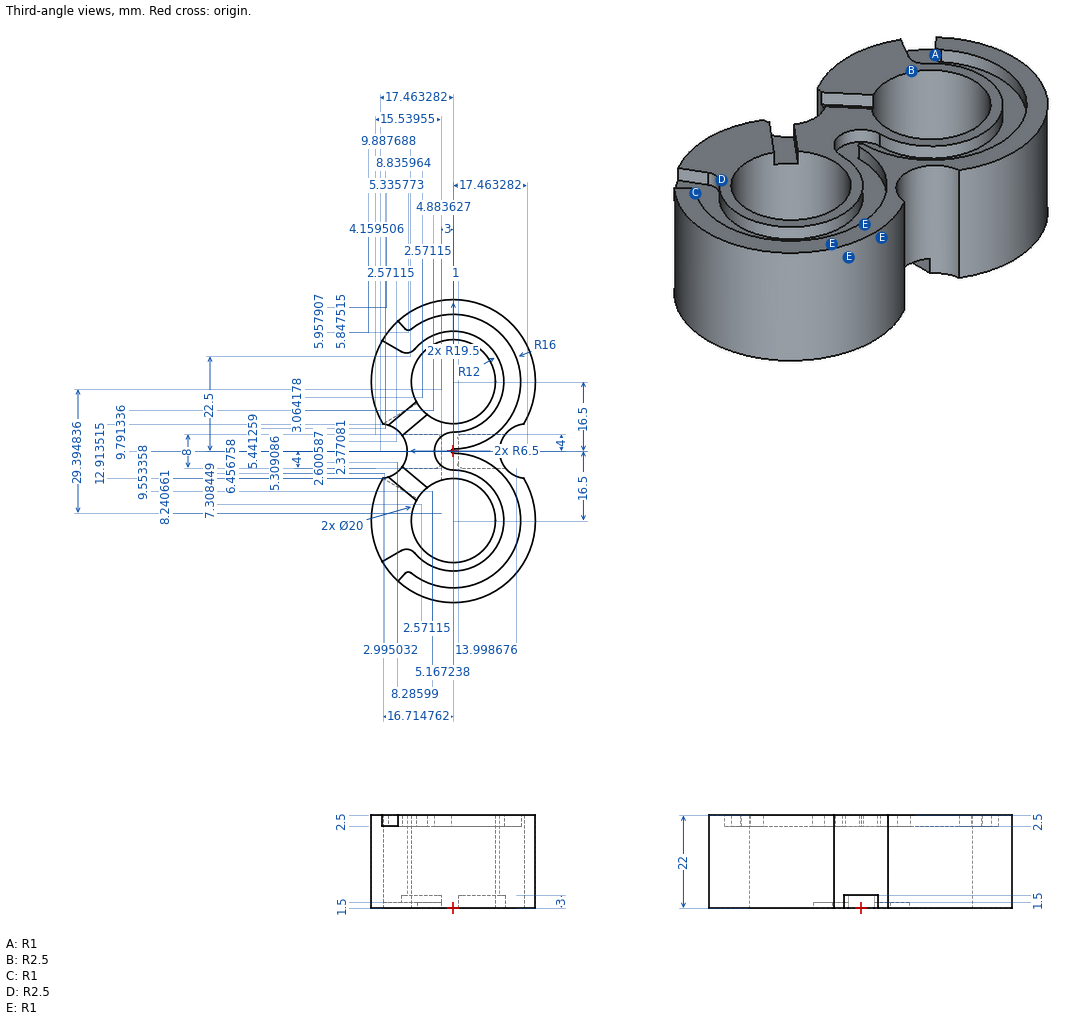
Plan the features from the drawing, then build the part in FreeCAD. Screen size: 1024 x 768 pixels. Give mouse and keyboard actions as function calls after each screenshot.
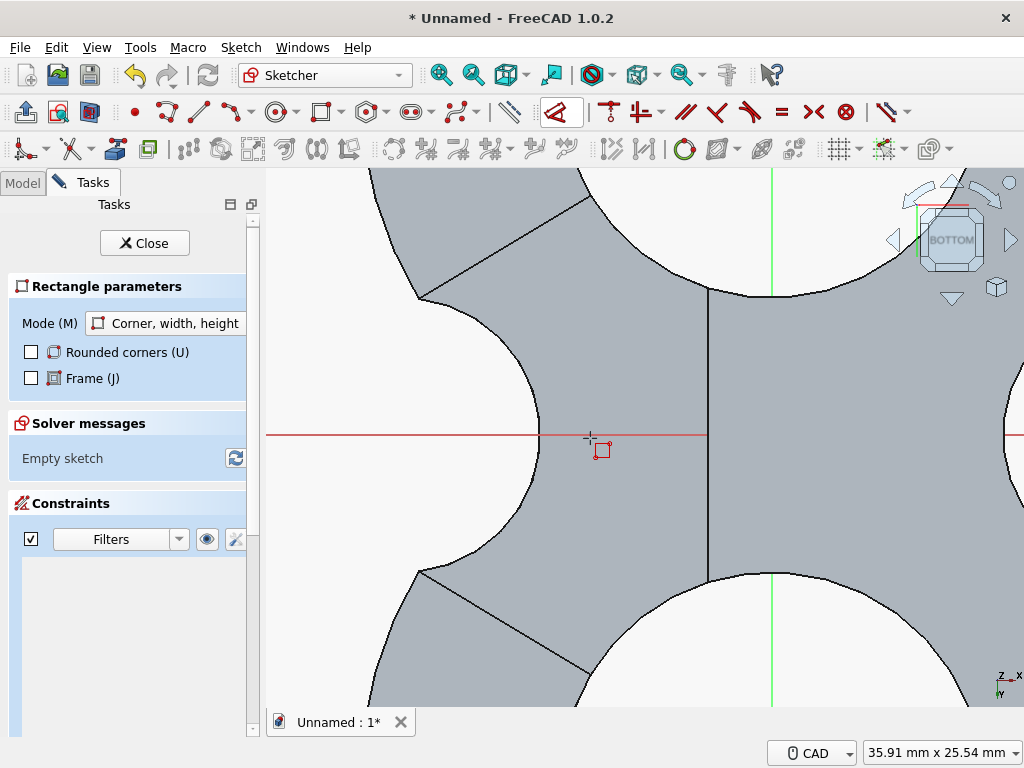
click(380, 351)
move(708, 520)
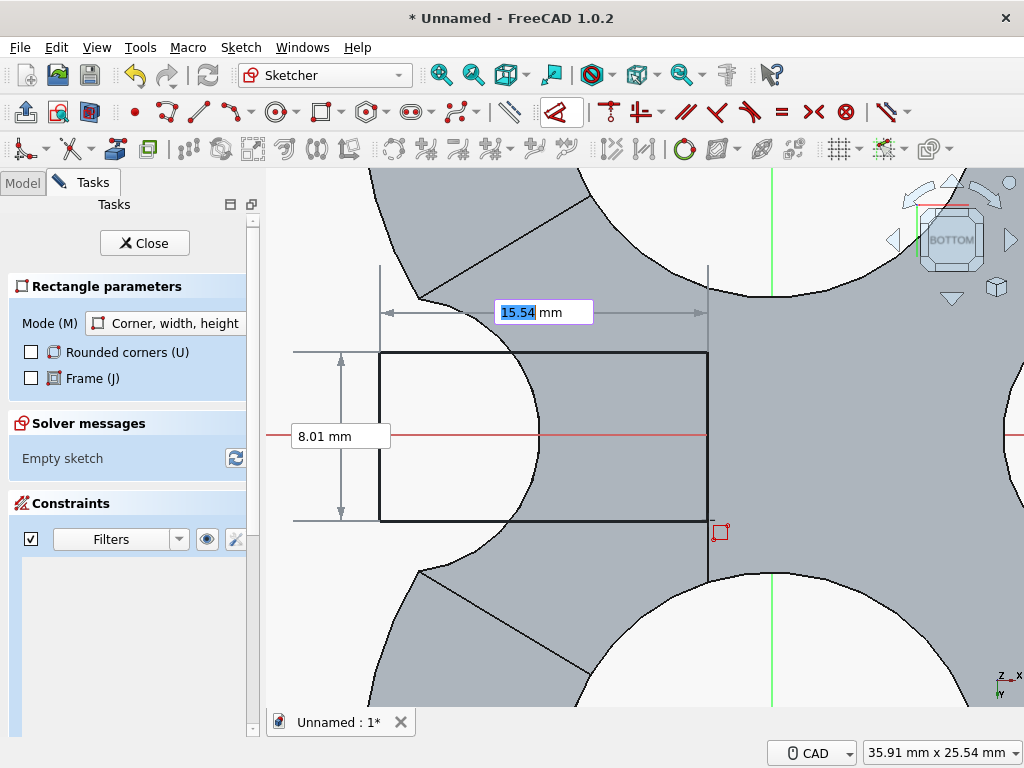
text(15.53955)
key(Tab)
text(8)
key(Return)
key(Escape)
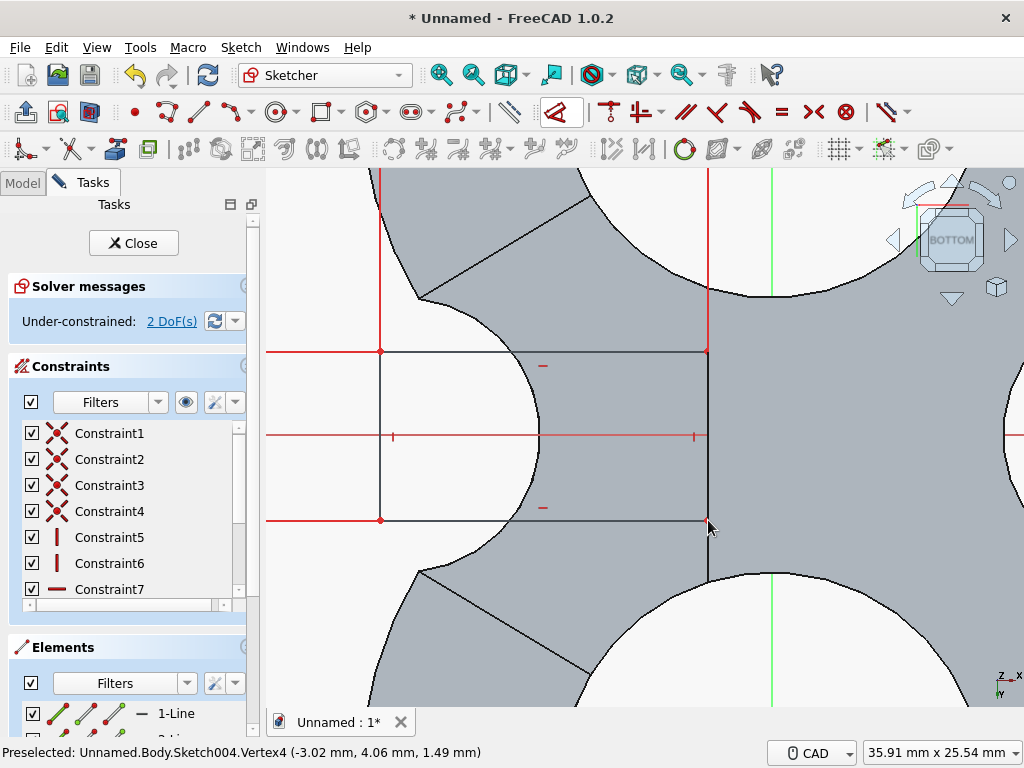
click(380, 352)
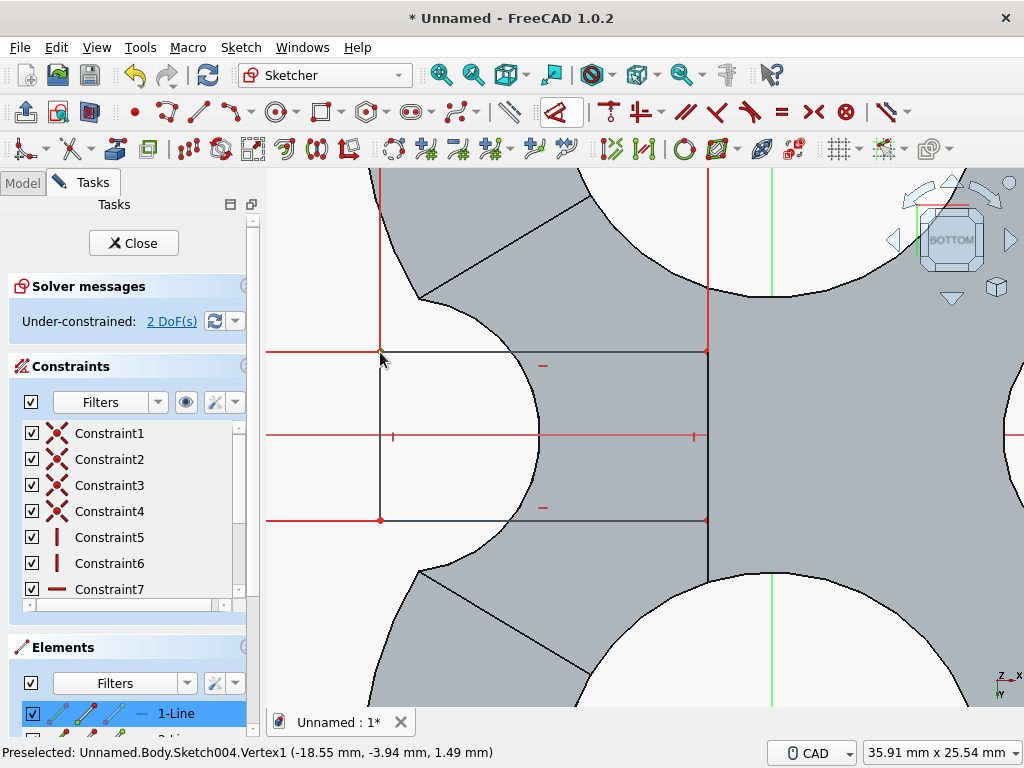
key(i)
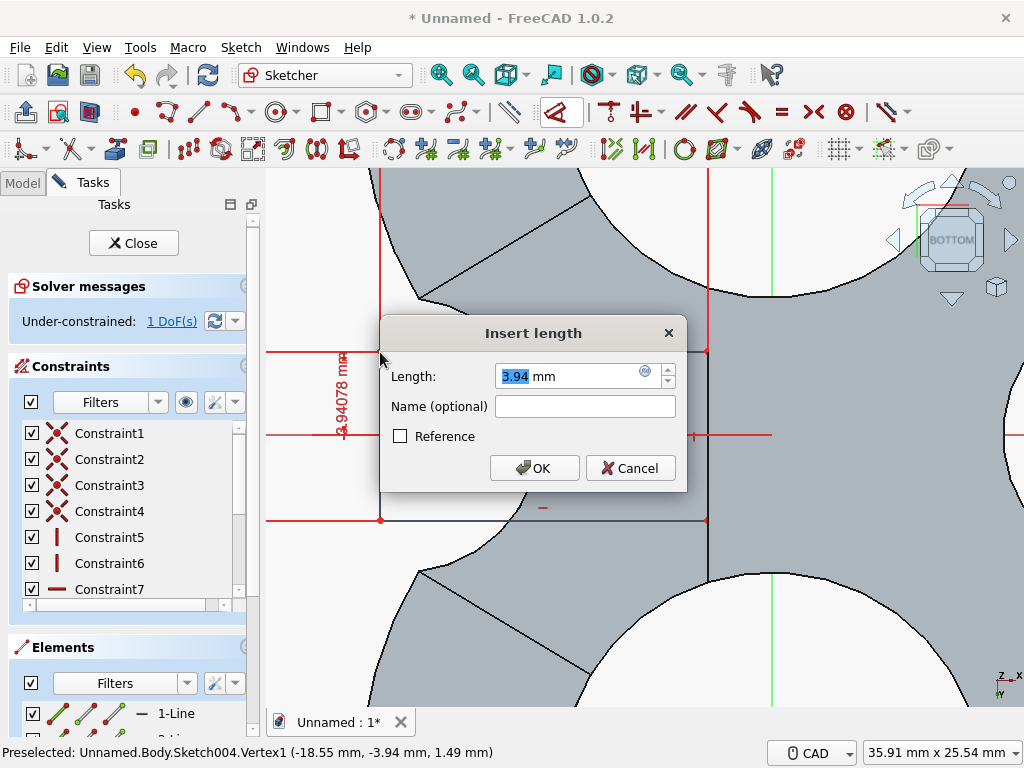
text(4)
key(Return)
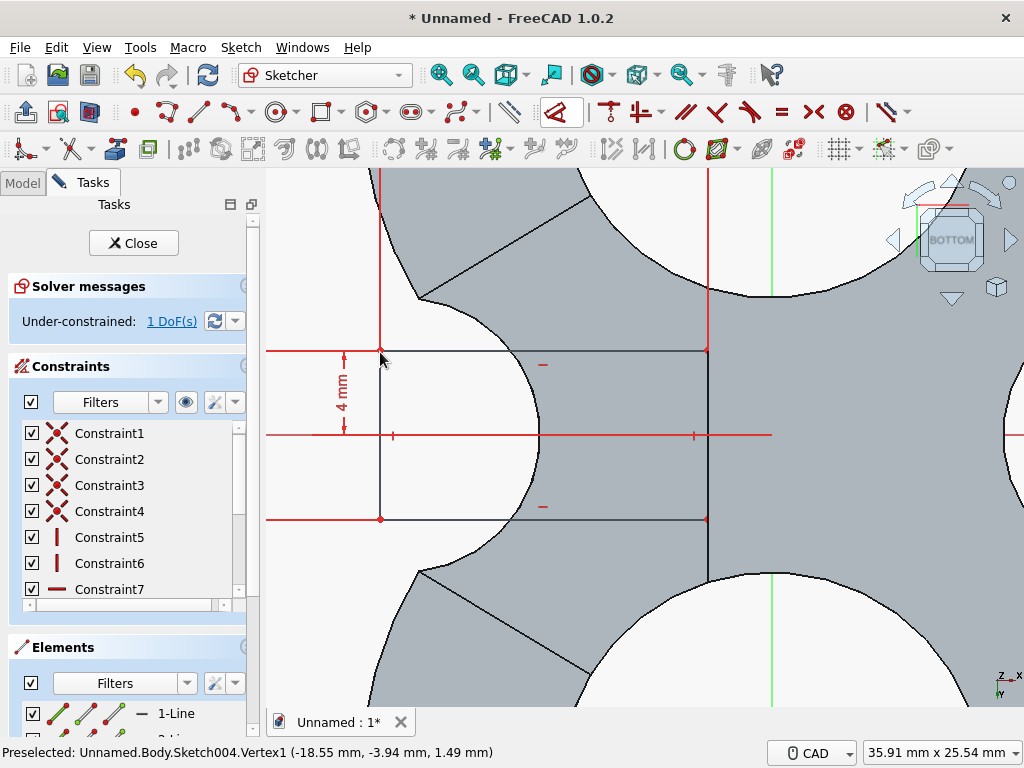
click(708, 520)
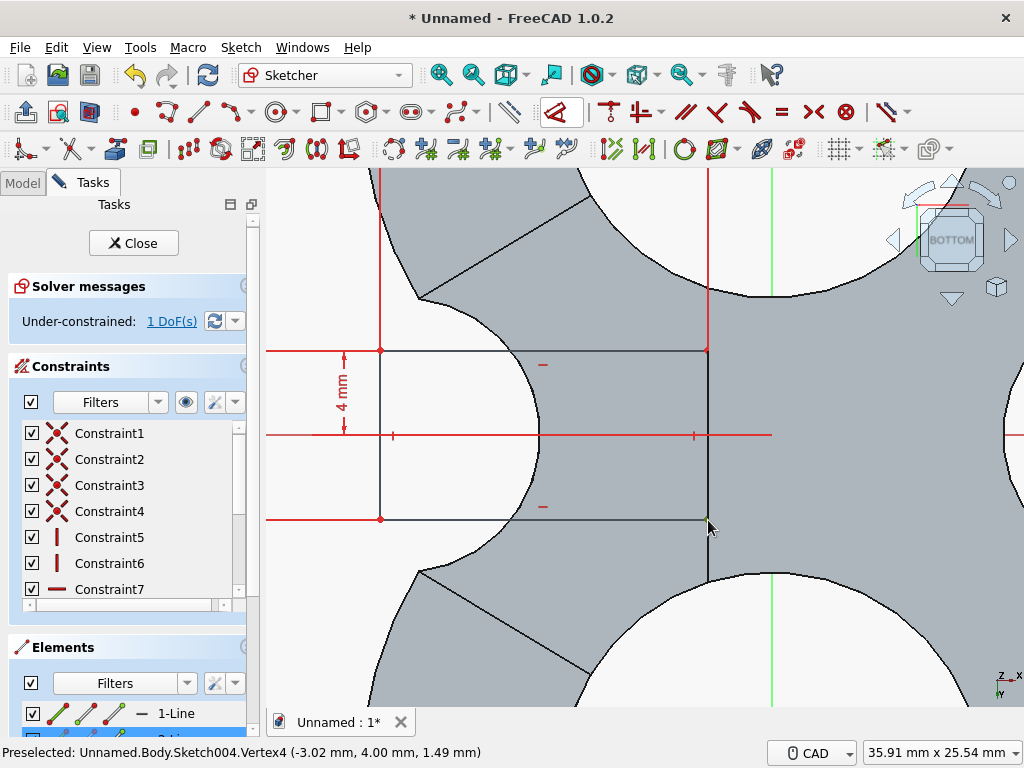
key(l)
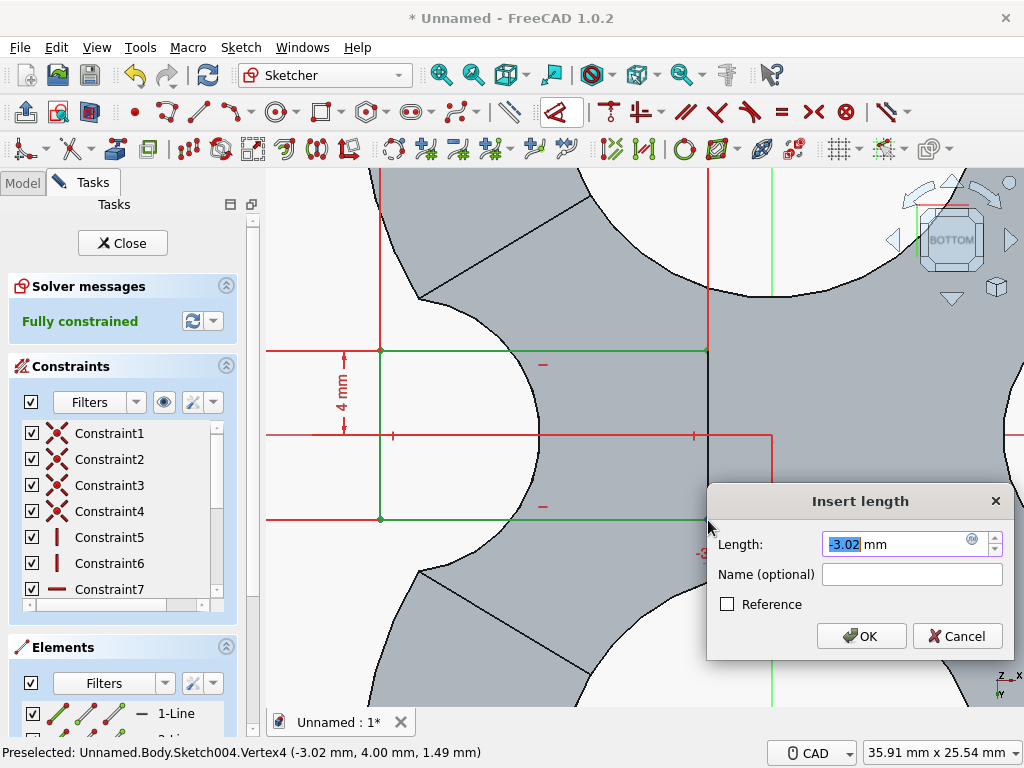
text(-3)
key(Return)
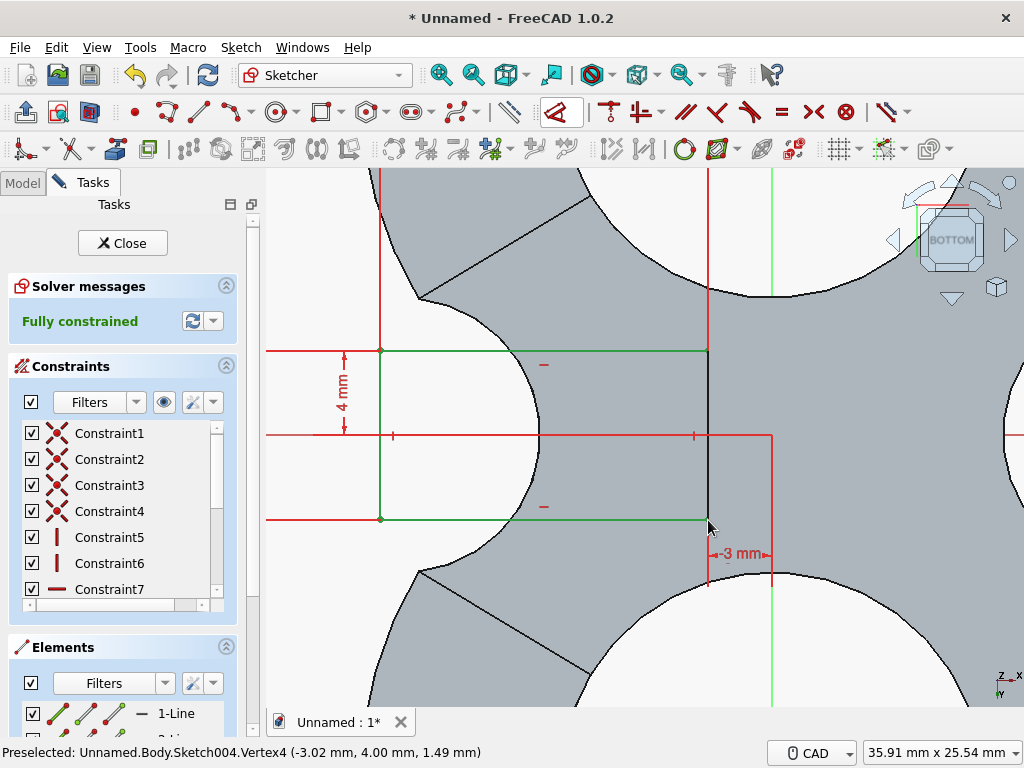
click(123, 243)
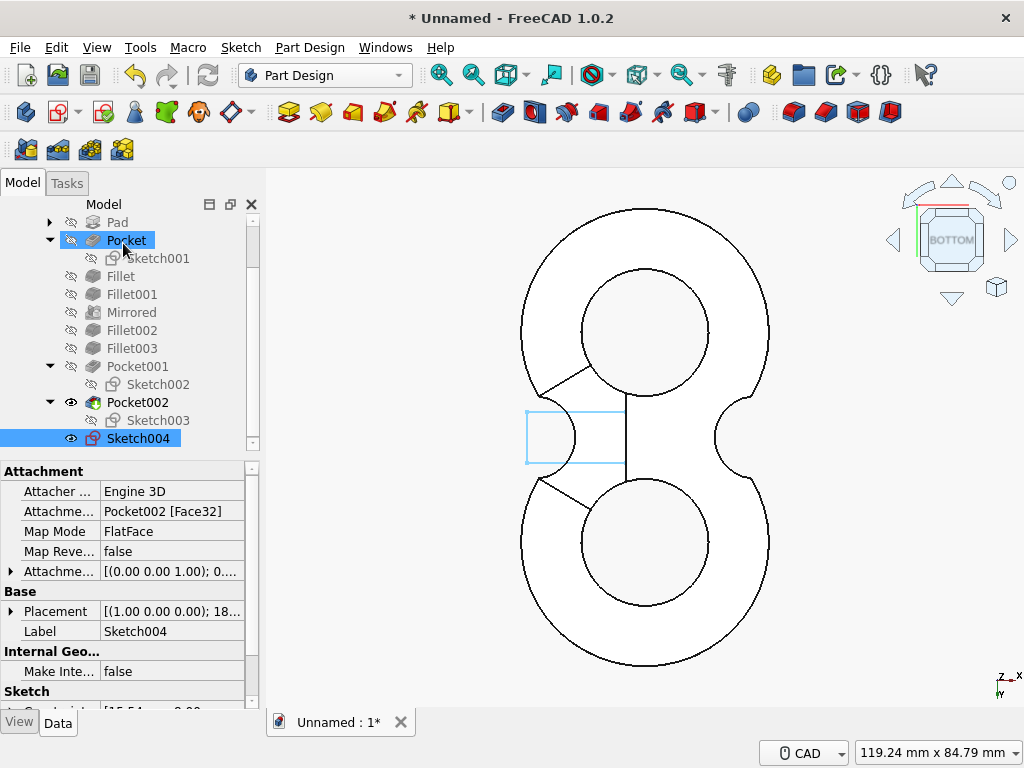
click(504, 112)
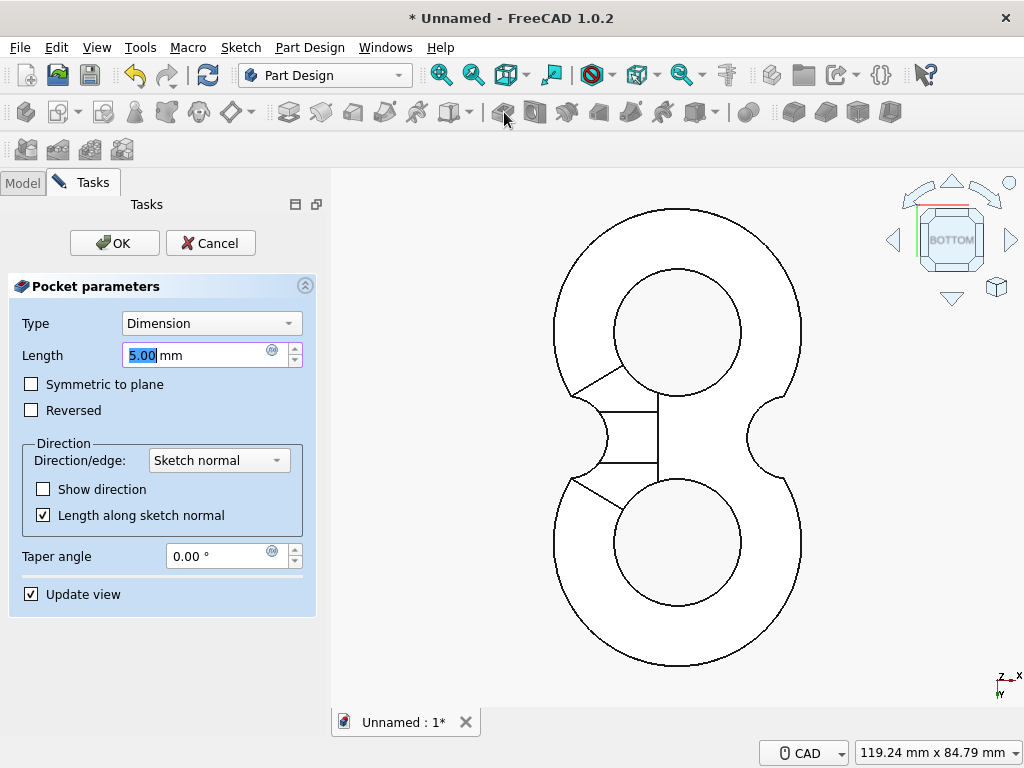
text(1.5)
key(Tab)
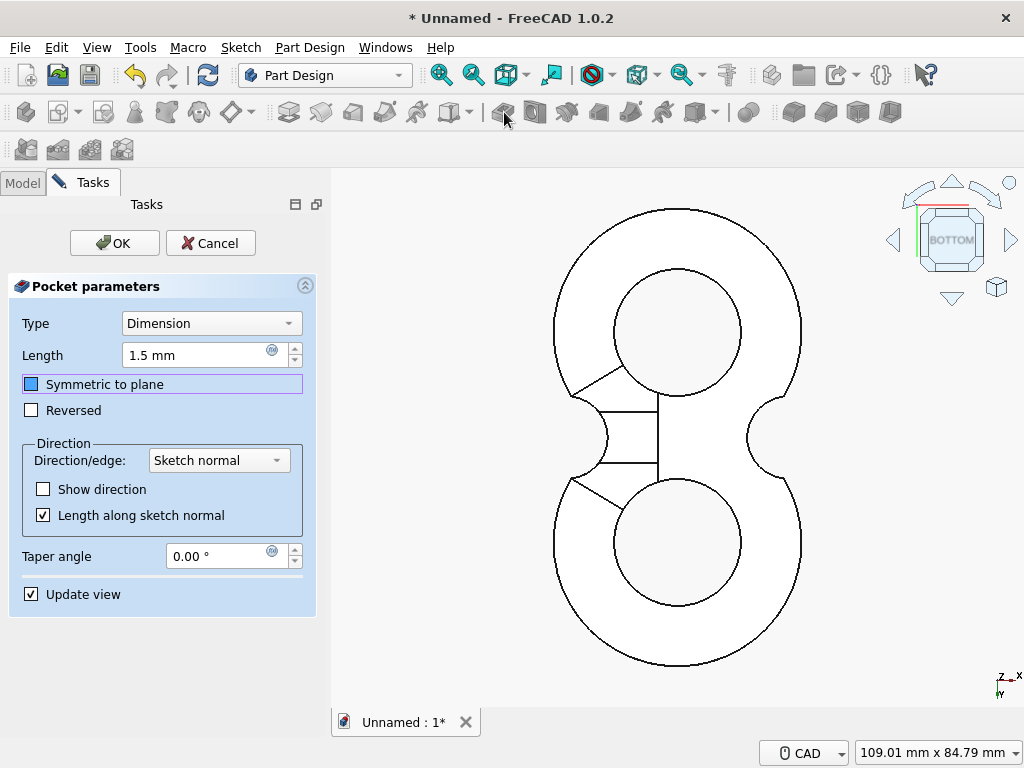
click(115, 243)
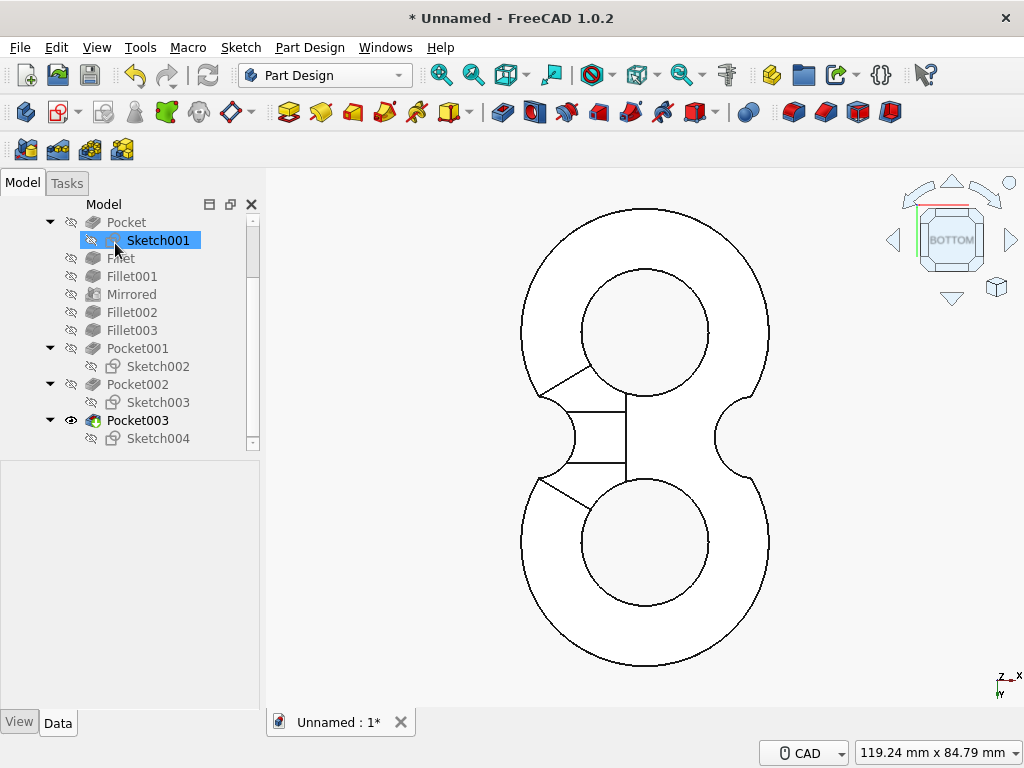
click(58, 112)